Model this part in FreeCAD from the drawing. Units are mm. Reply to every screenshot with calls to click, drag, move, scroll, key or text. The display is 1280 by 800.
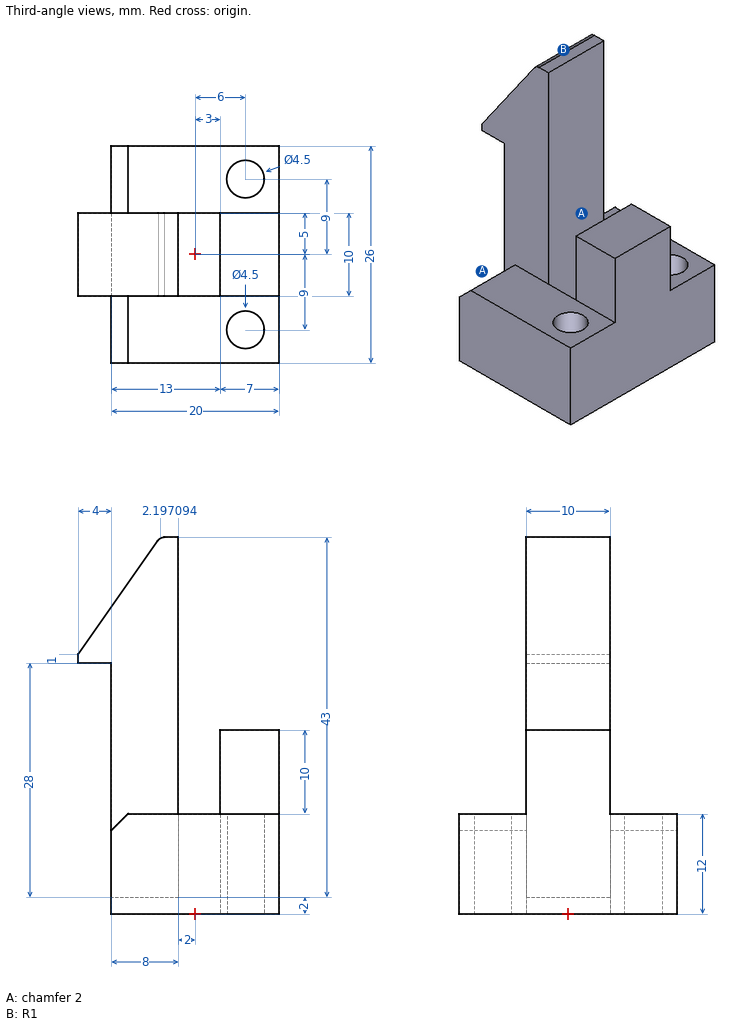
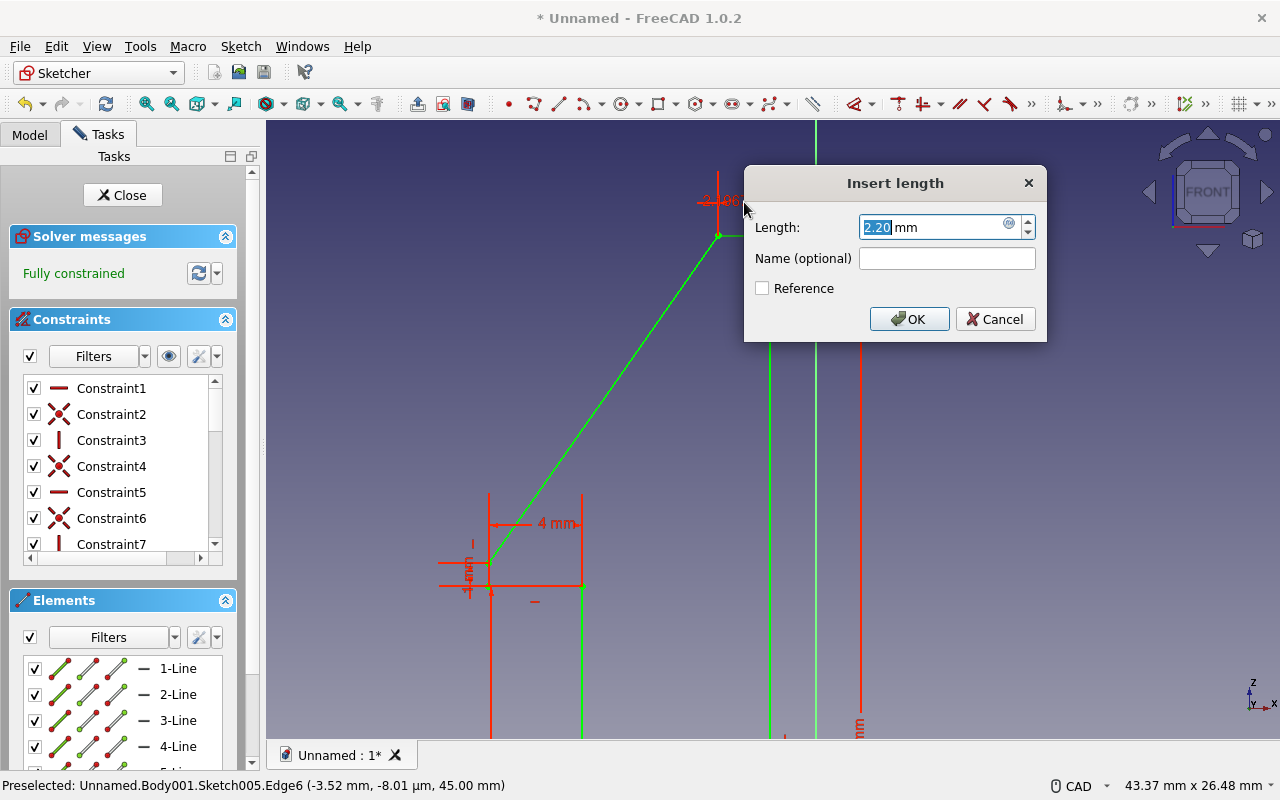
text(2.197094)
key(Return)
key(Escape)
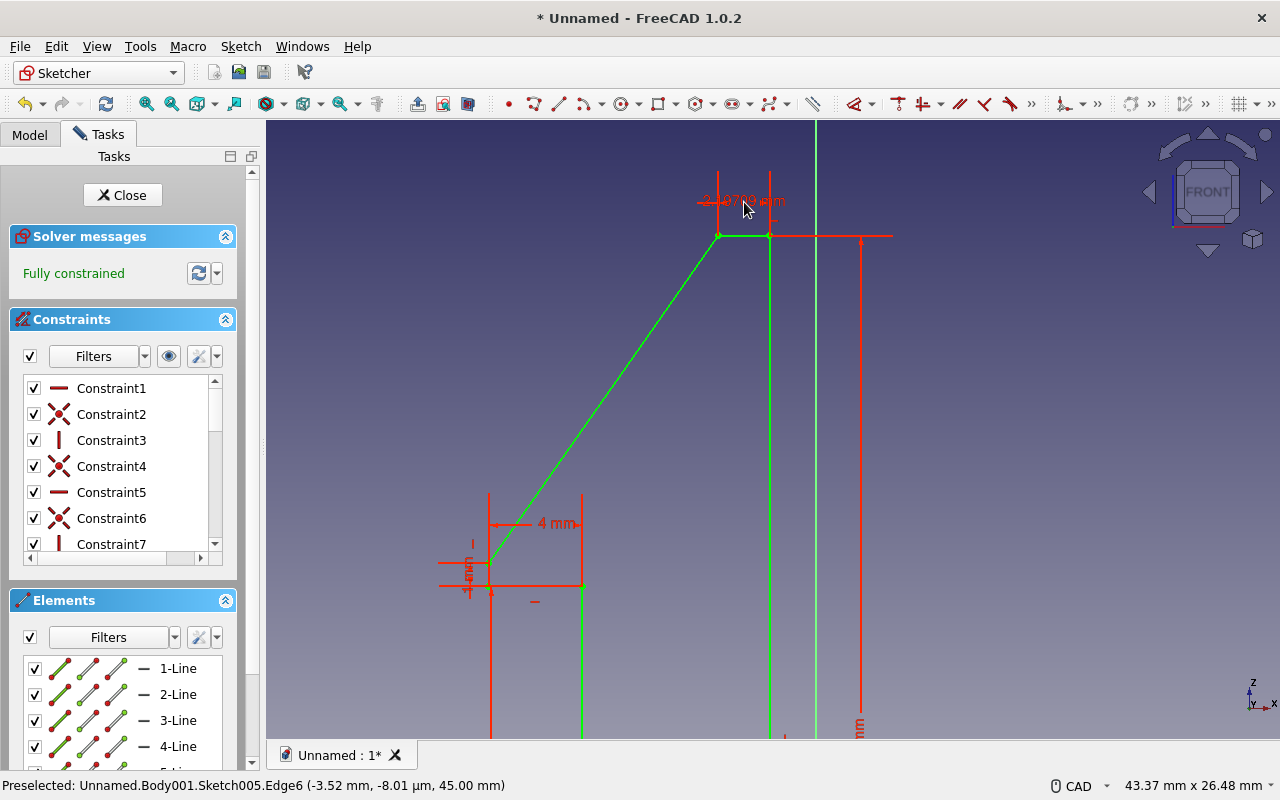
click(123, 195)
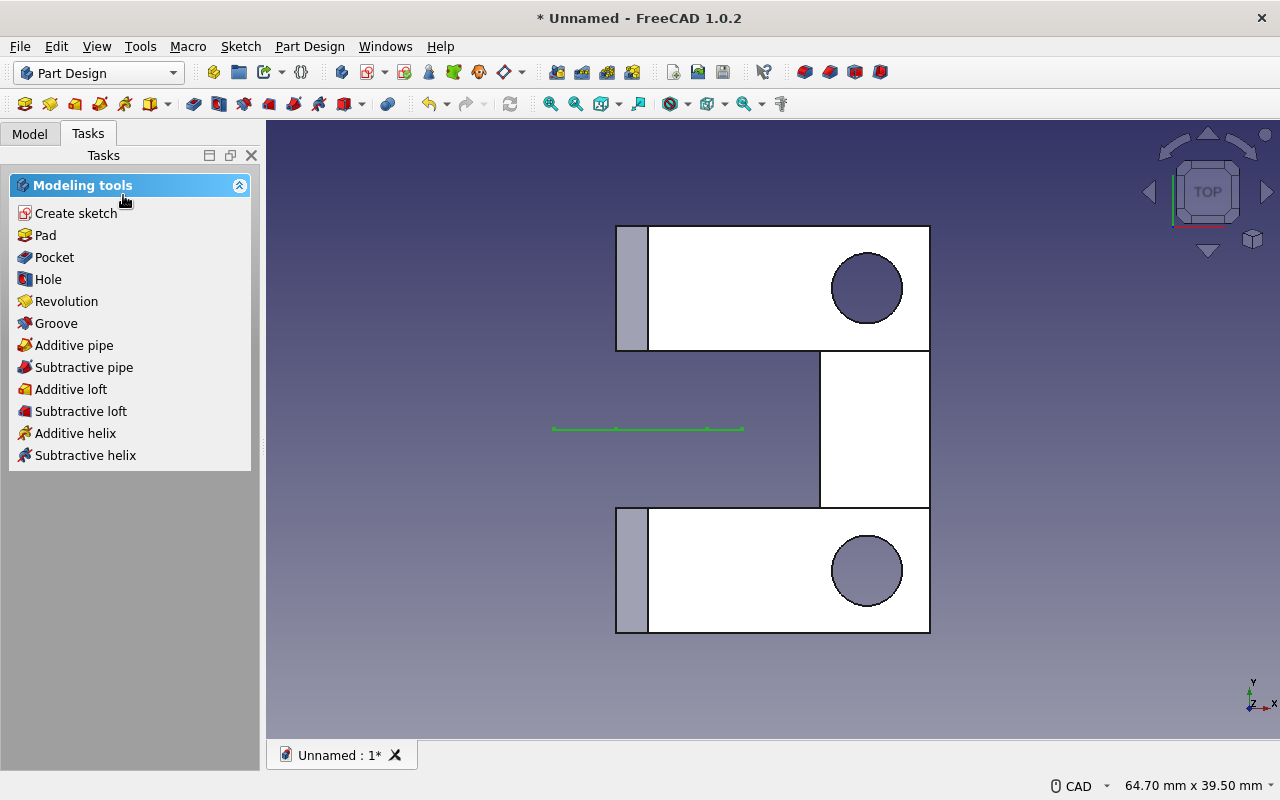
click(25, 104)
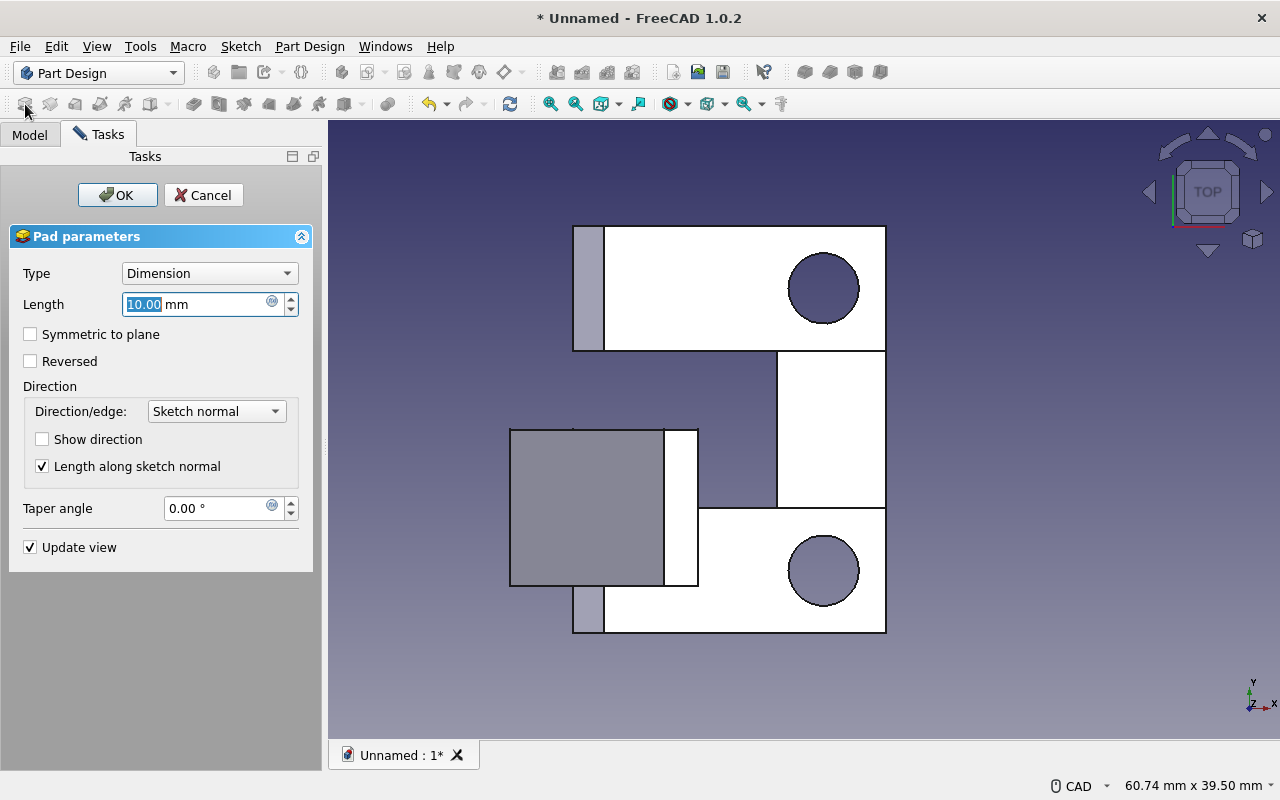
text(10)
key(Tab)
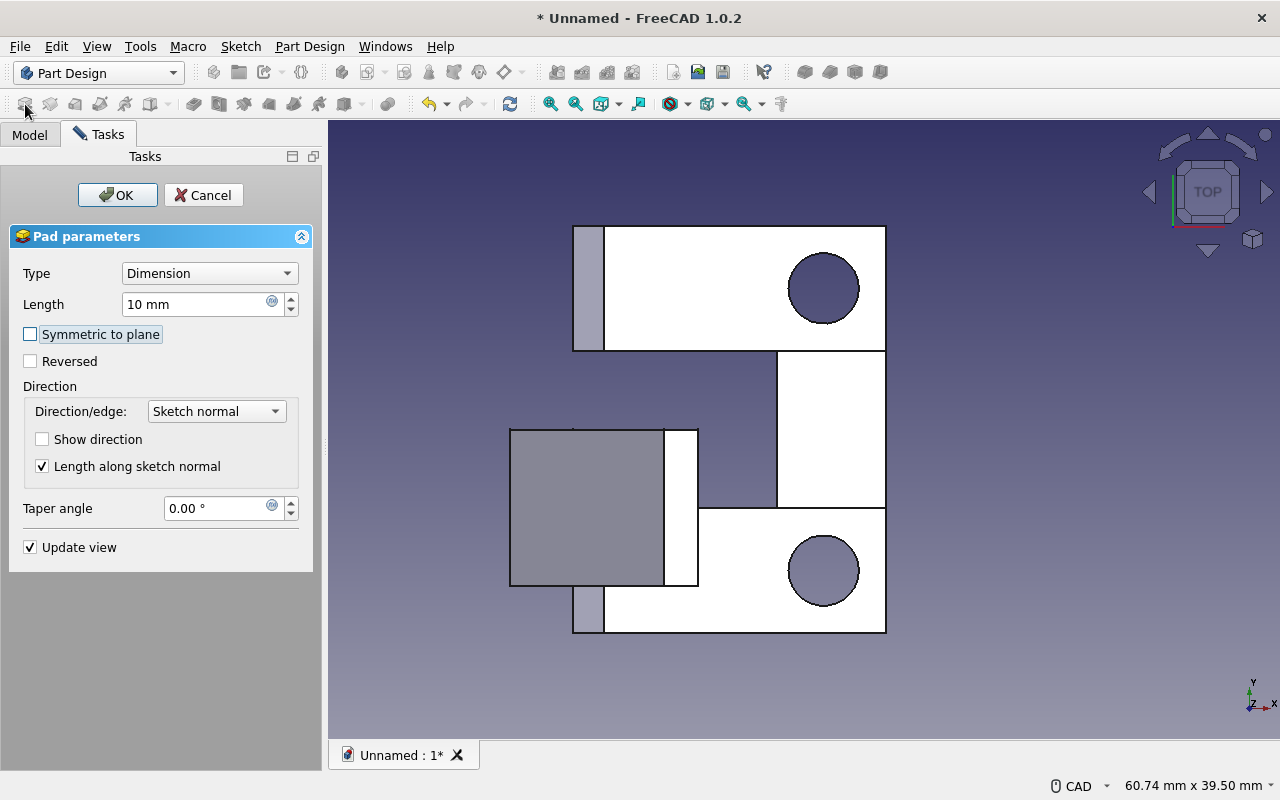
click(31, 334)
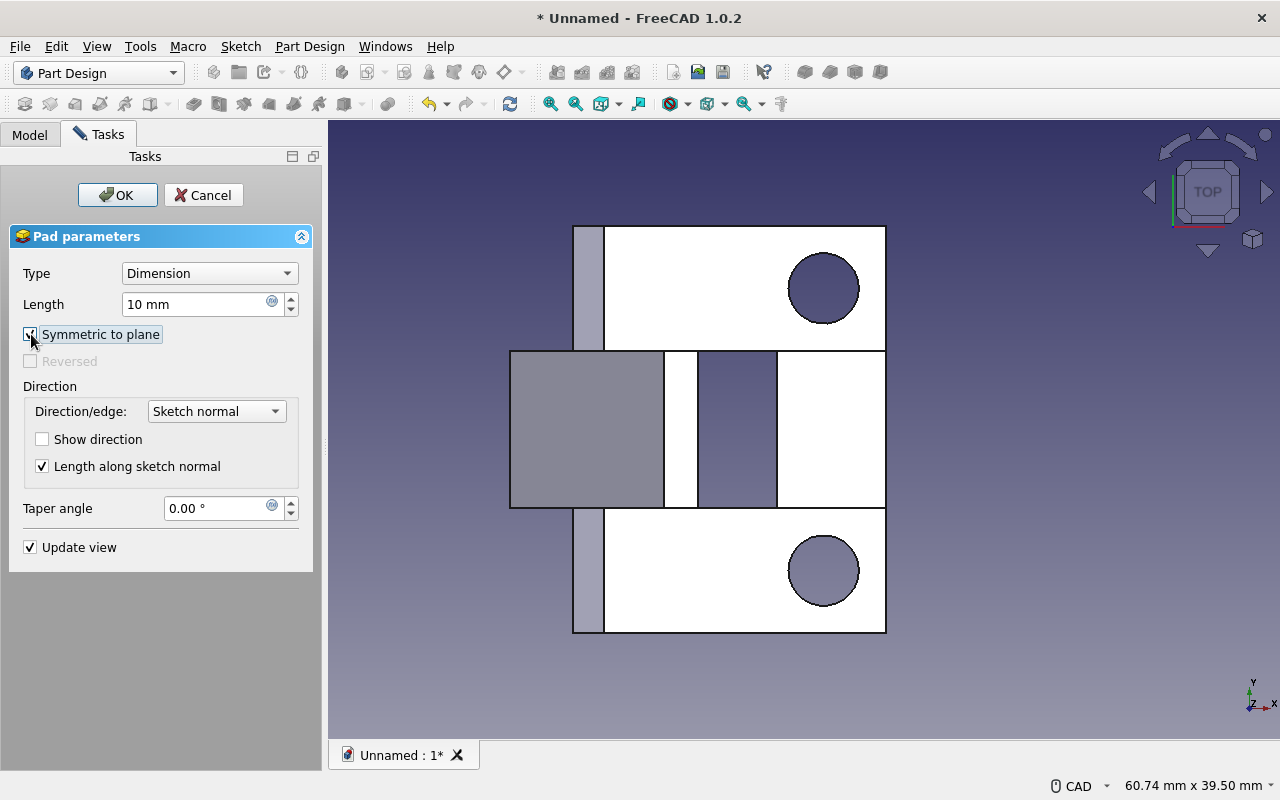
click(118, 195)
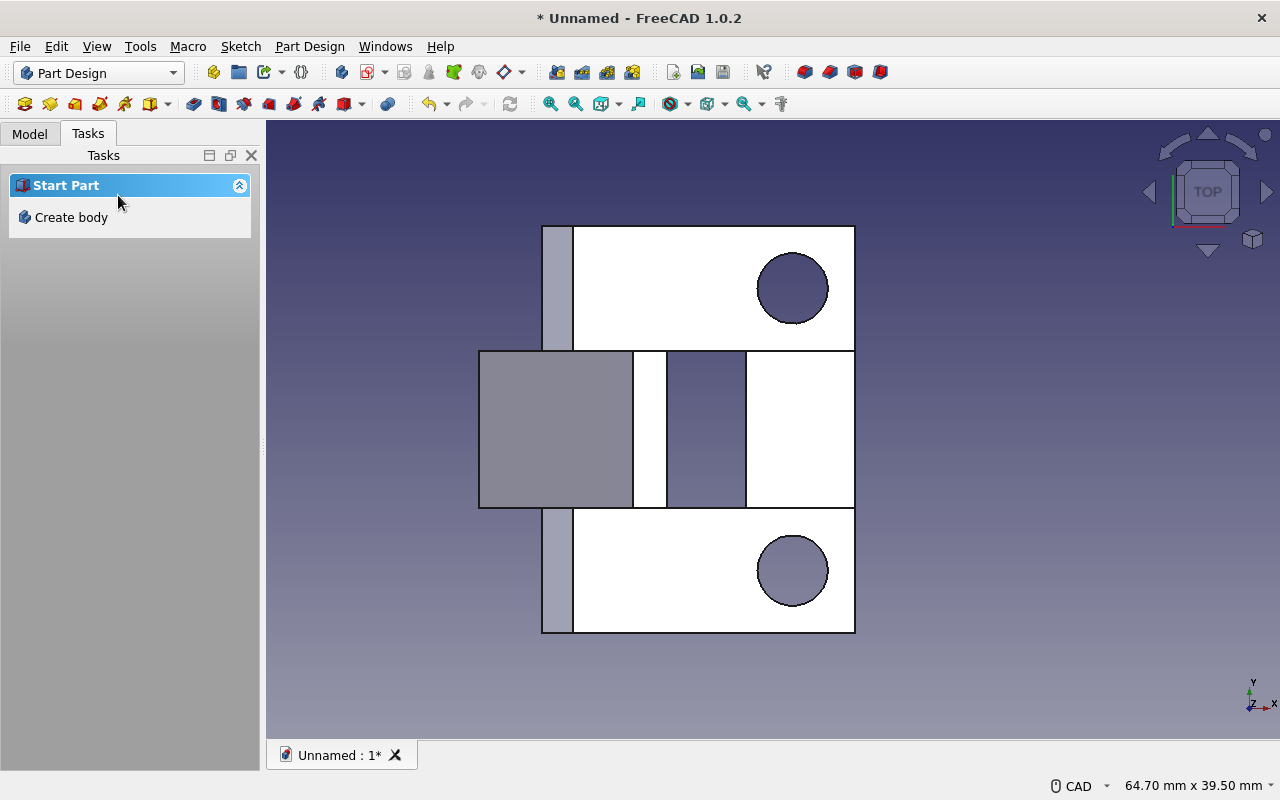
click(551, 104)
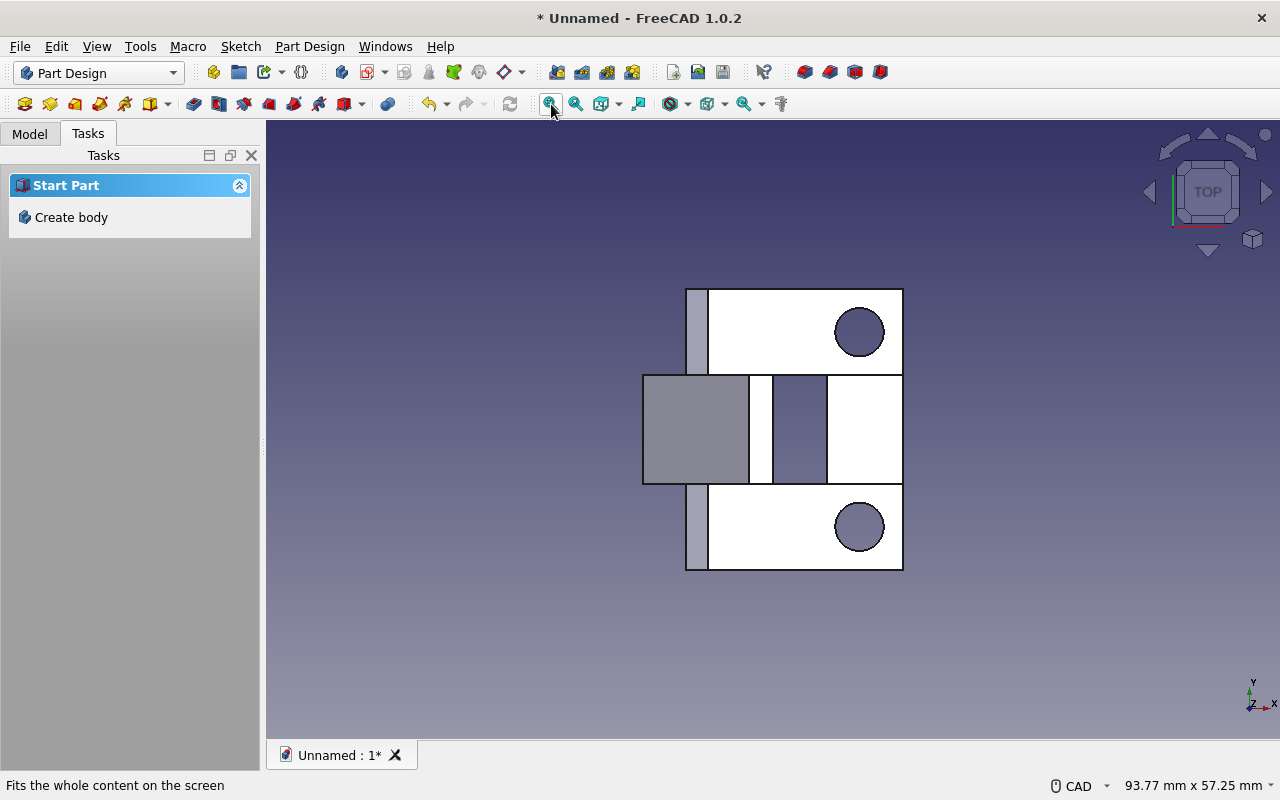
click(749, 428)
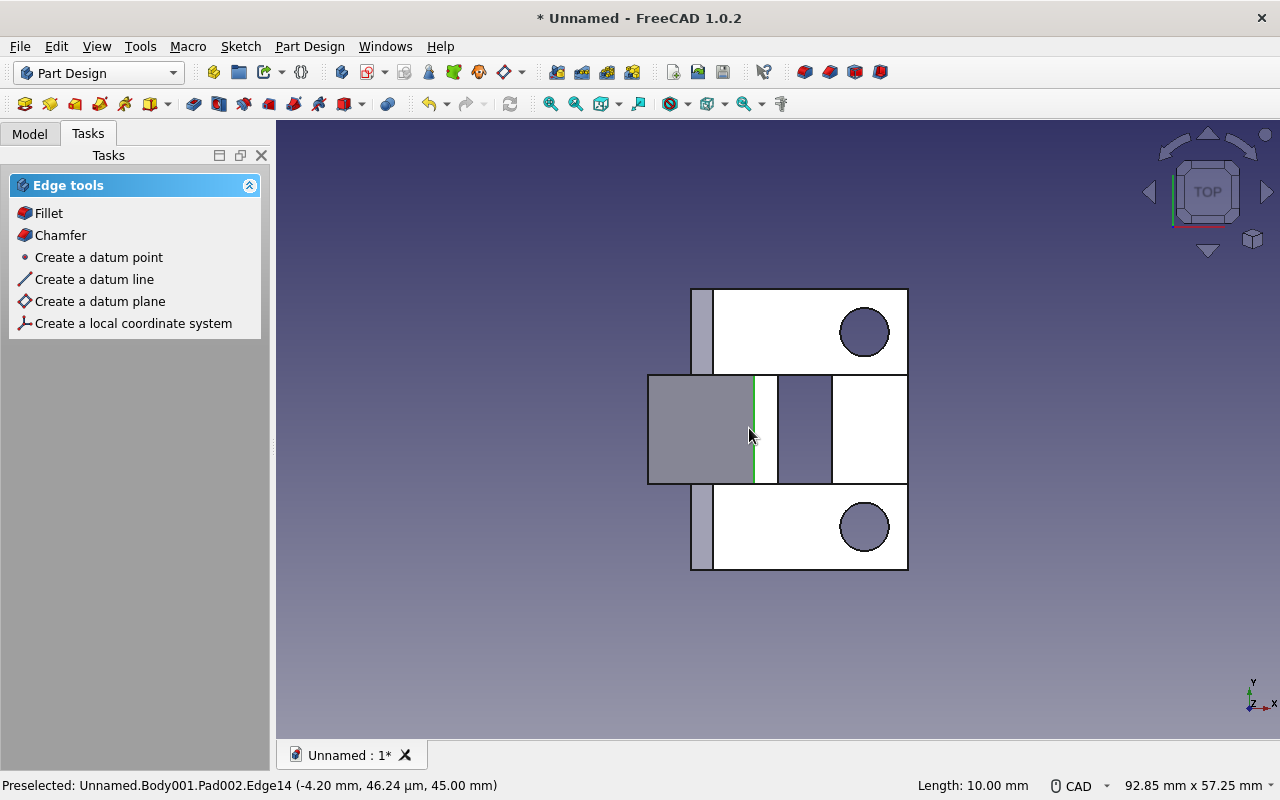
click(805, 72)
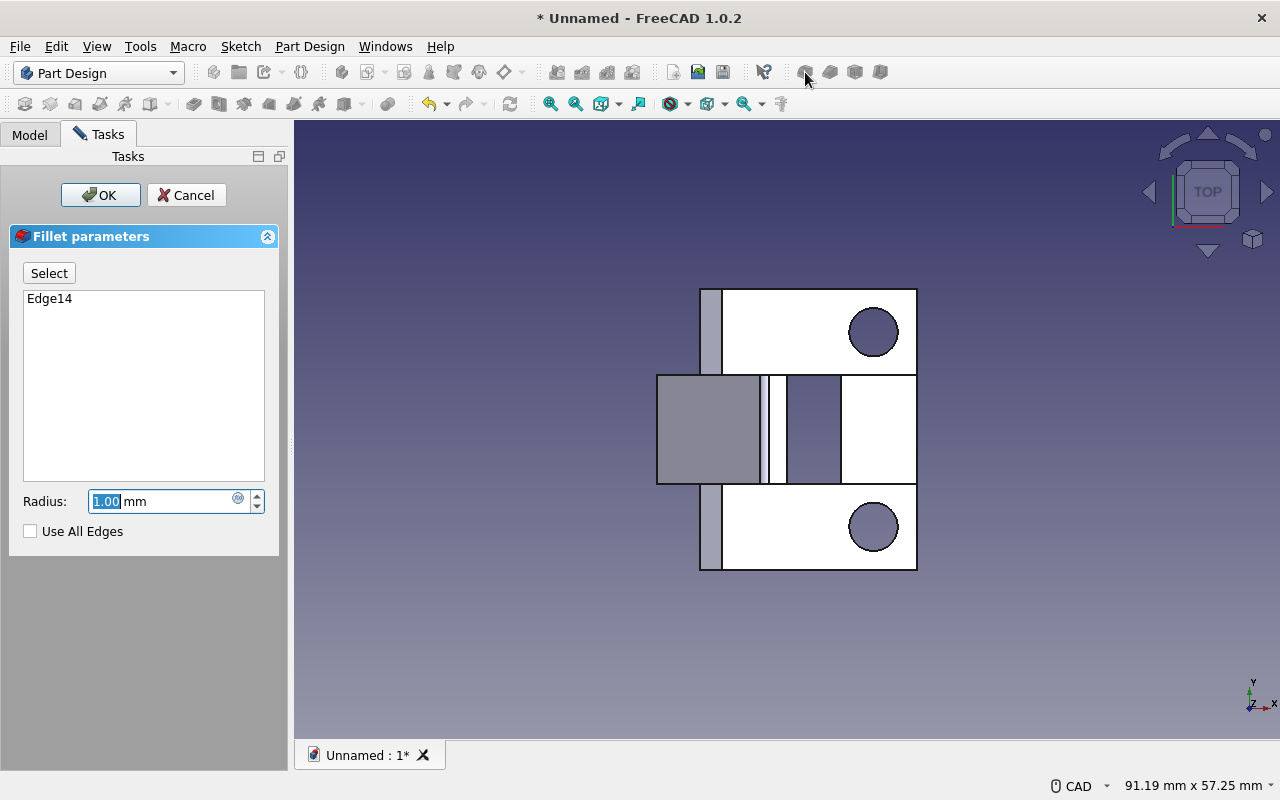
text(1)
key(Tab)